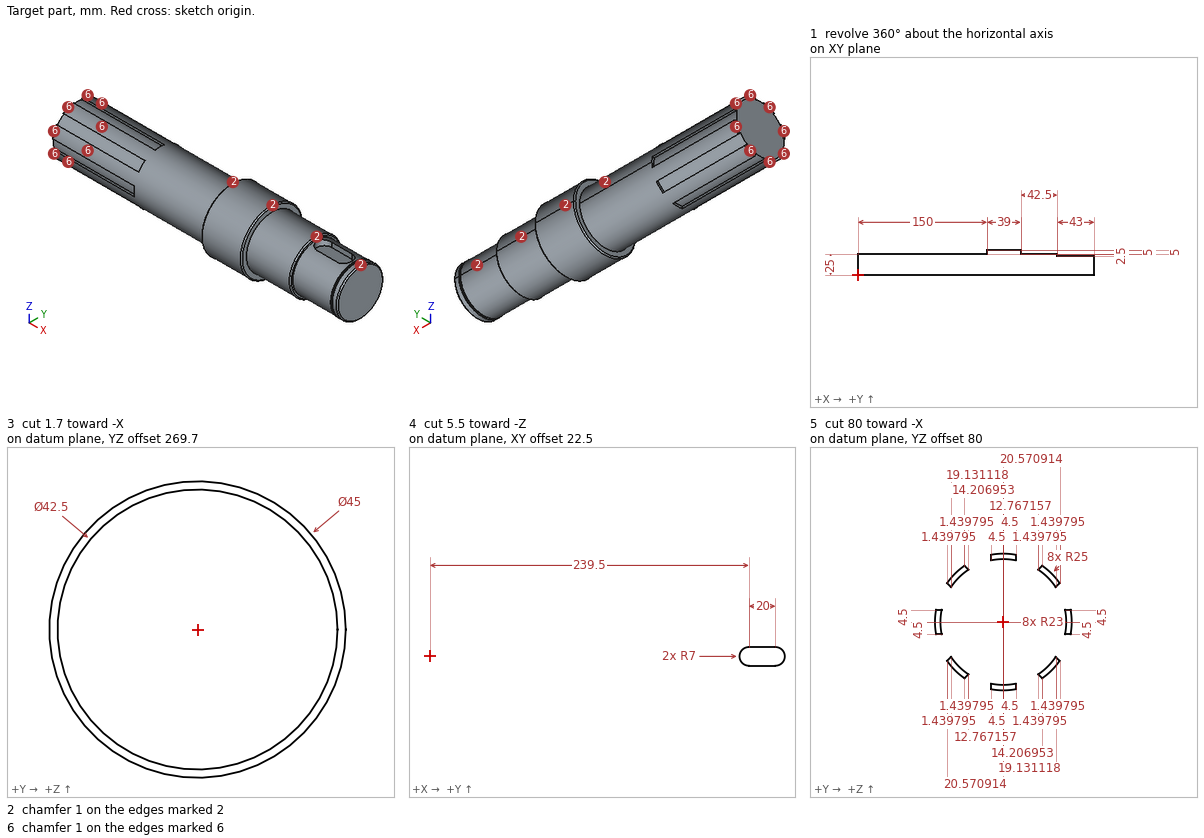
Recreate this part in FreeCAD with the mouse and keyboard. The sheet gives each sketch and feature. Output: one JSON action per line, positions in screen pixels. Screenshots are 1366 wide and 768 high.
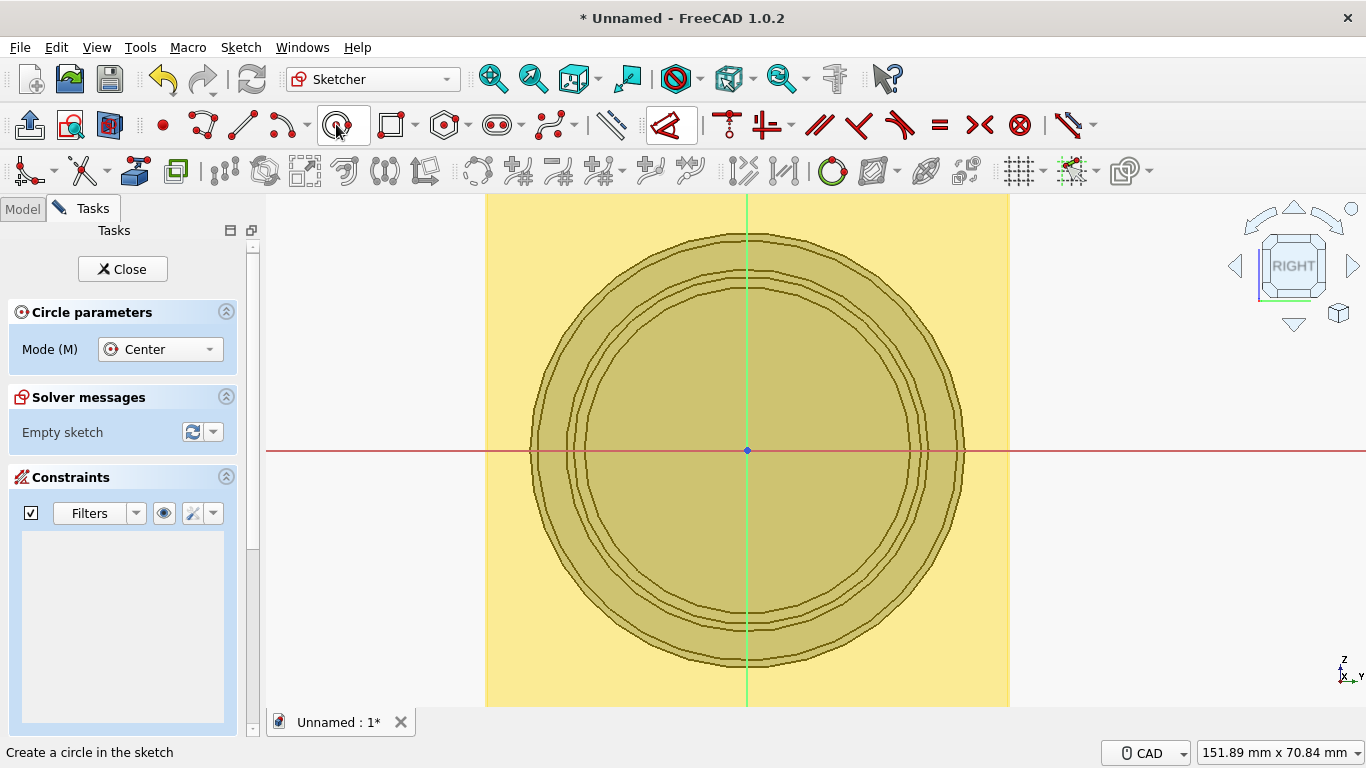
{"action": "left_click", "coordinate": [747, 450]}
{"action": "mouse_move", "coordinate": [863, 335]}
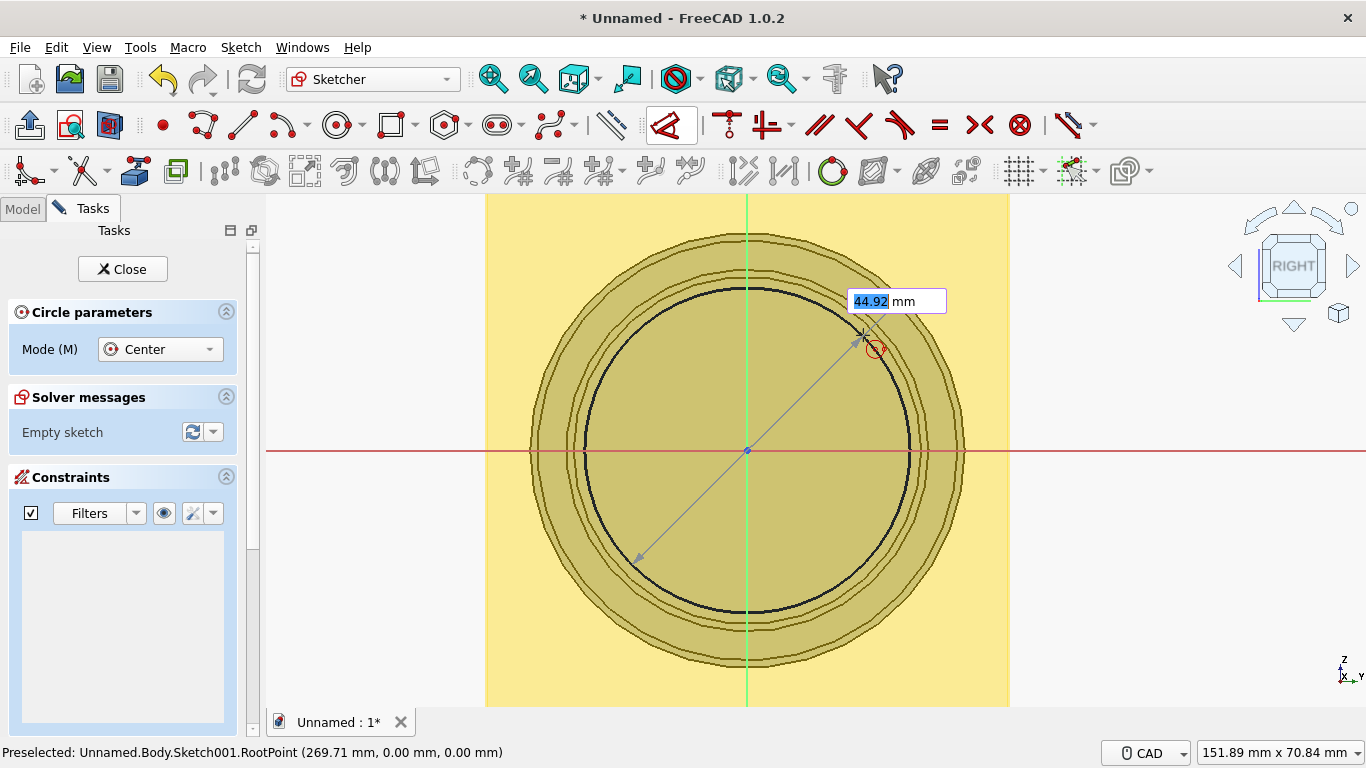
{"action": "type", "text": "45"}
{"action": "key", "text": "Return"}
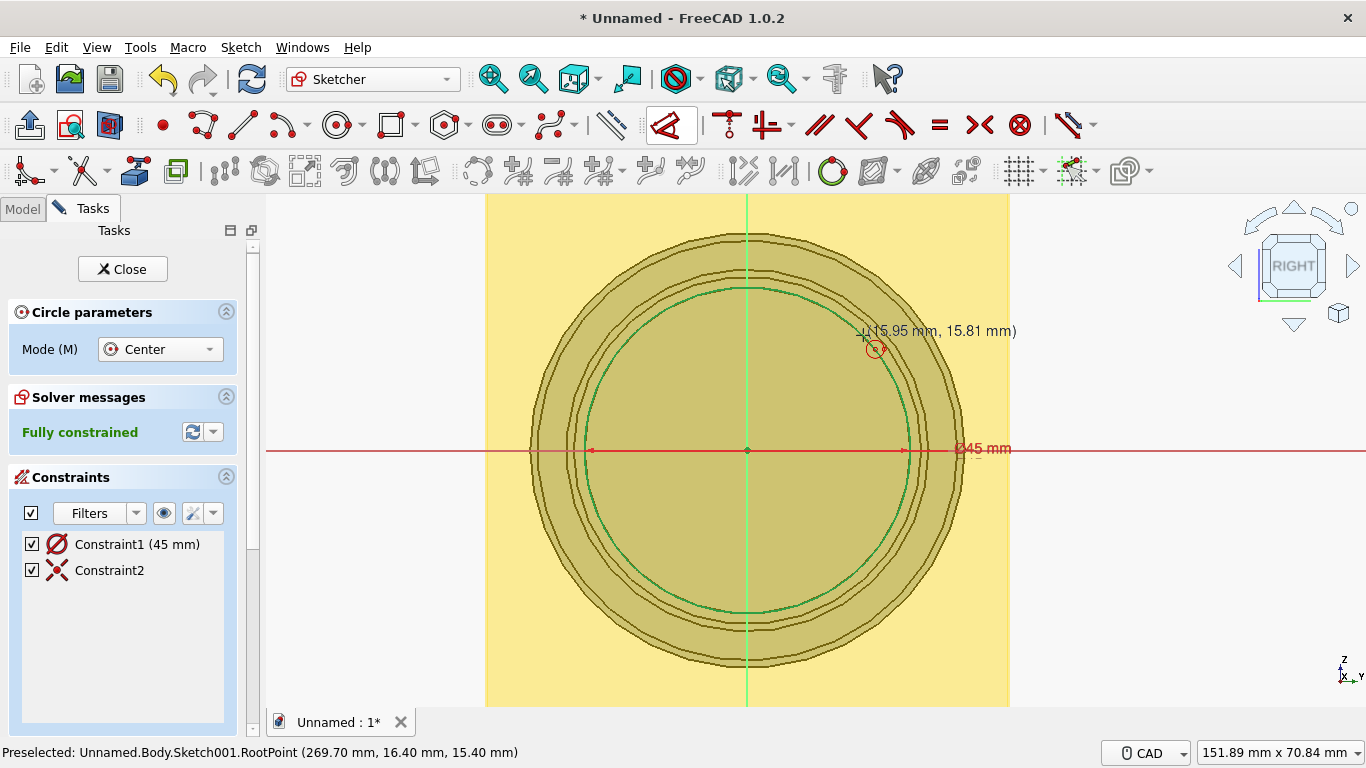
{"action": "left_click", "coordinate": [747, 450]}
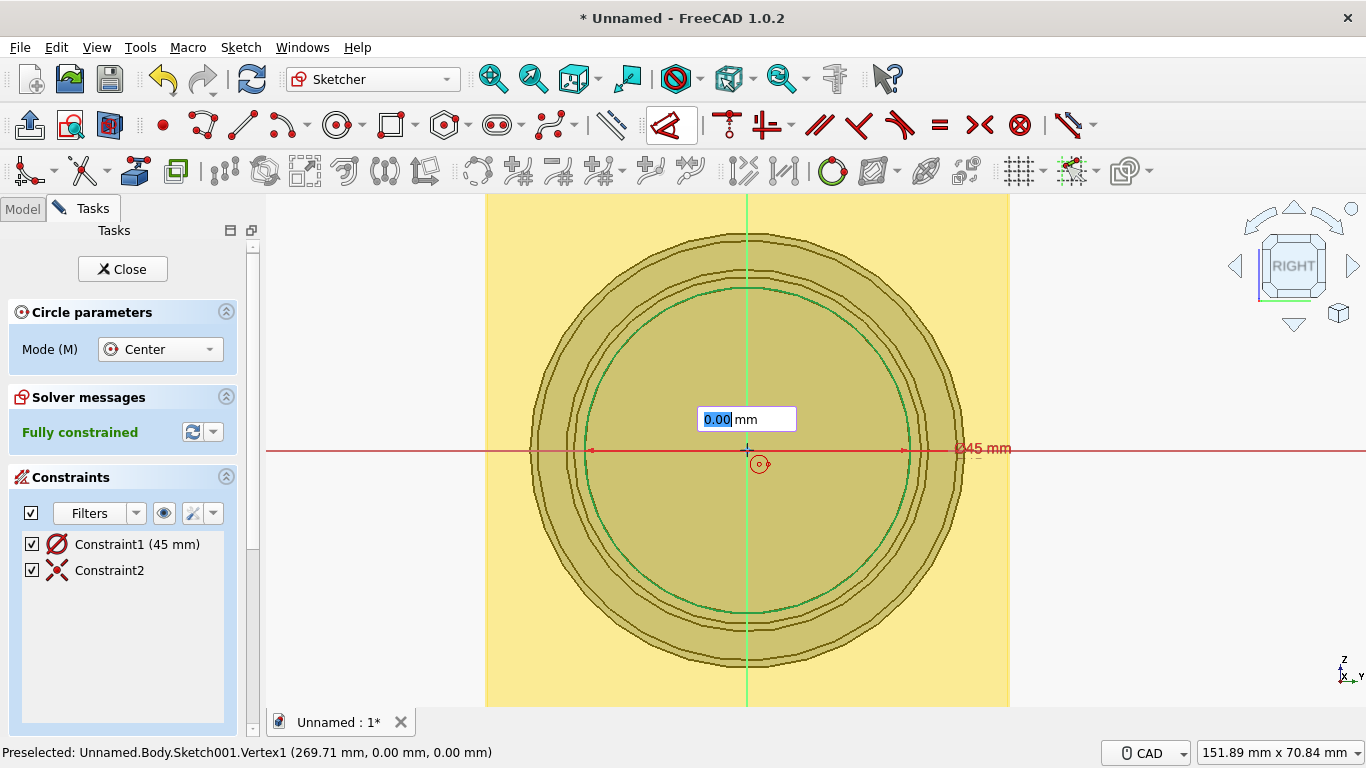
{"action": "scroll", "coordinate": [856, 342], "scroll_direction": "up", "scroll_amount": 3}
{"action": "mouse_move", "coordinate": [856, 341]}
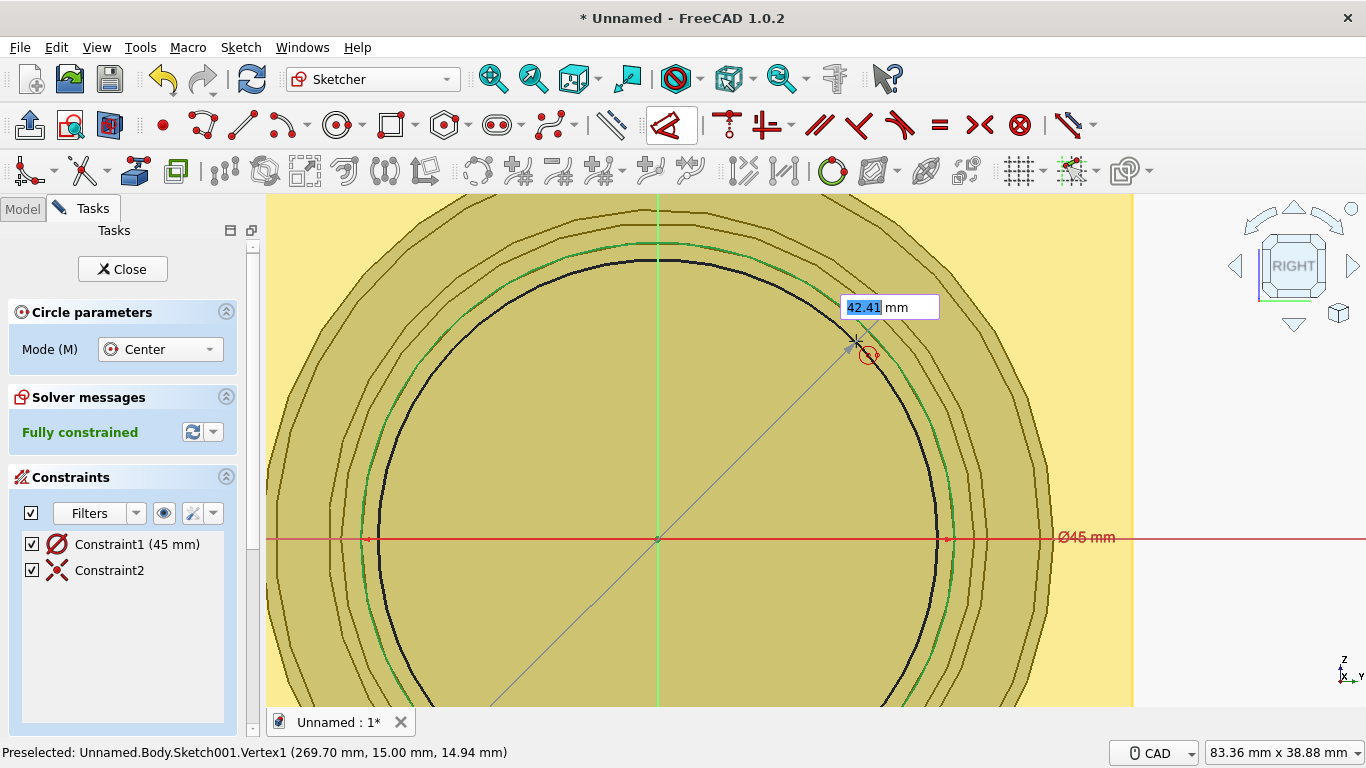
{"action": "type", "text": "42.5"}
{"action": "key", "text": "Return"}
{"action": "key", "text": "Escape"}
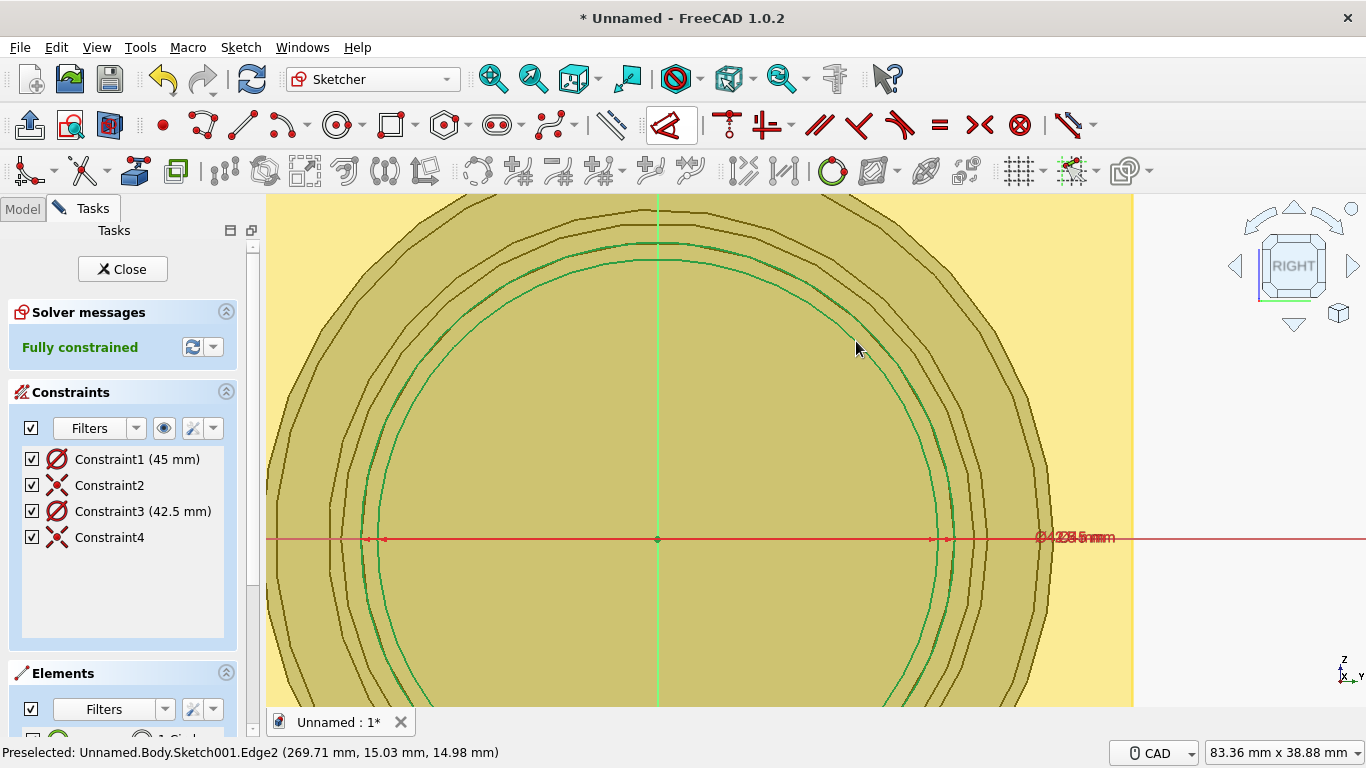
{"action": "left_click", "coordinate": [123, 269]}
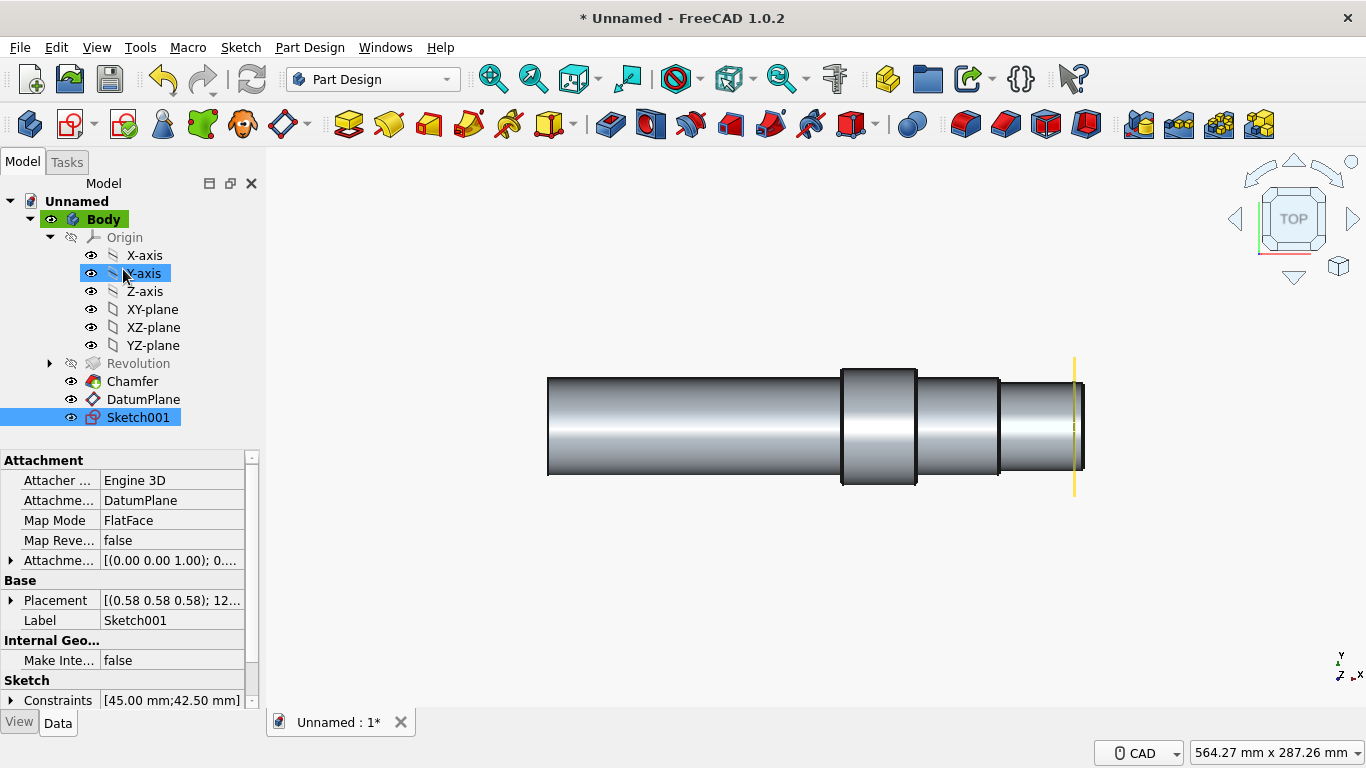
{"action": "left_click", "coordinate": [612, 124]}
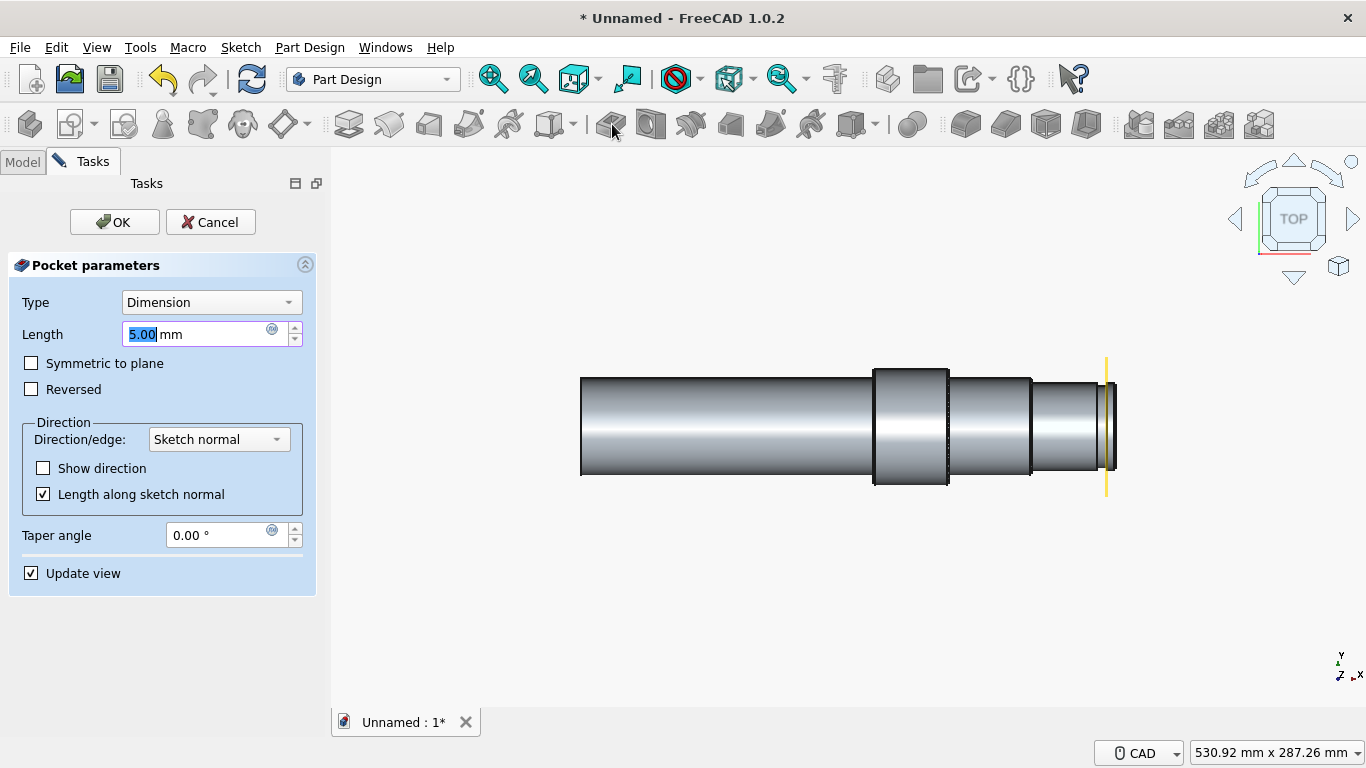
{"action": "type", "text": "1.7"}
{"action": "key", "text": "Tab"}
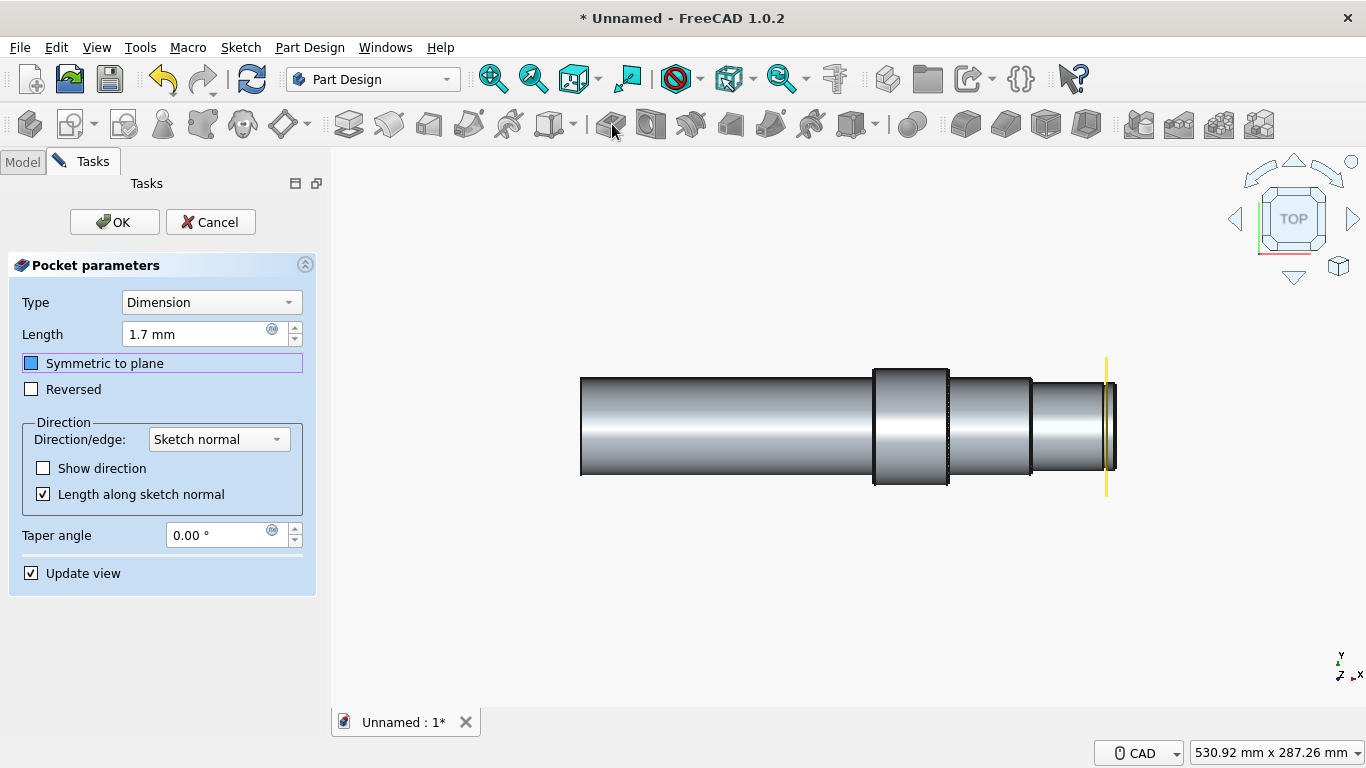
{"action": "left_click", "coordinate": [115, 222]}